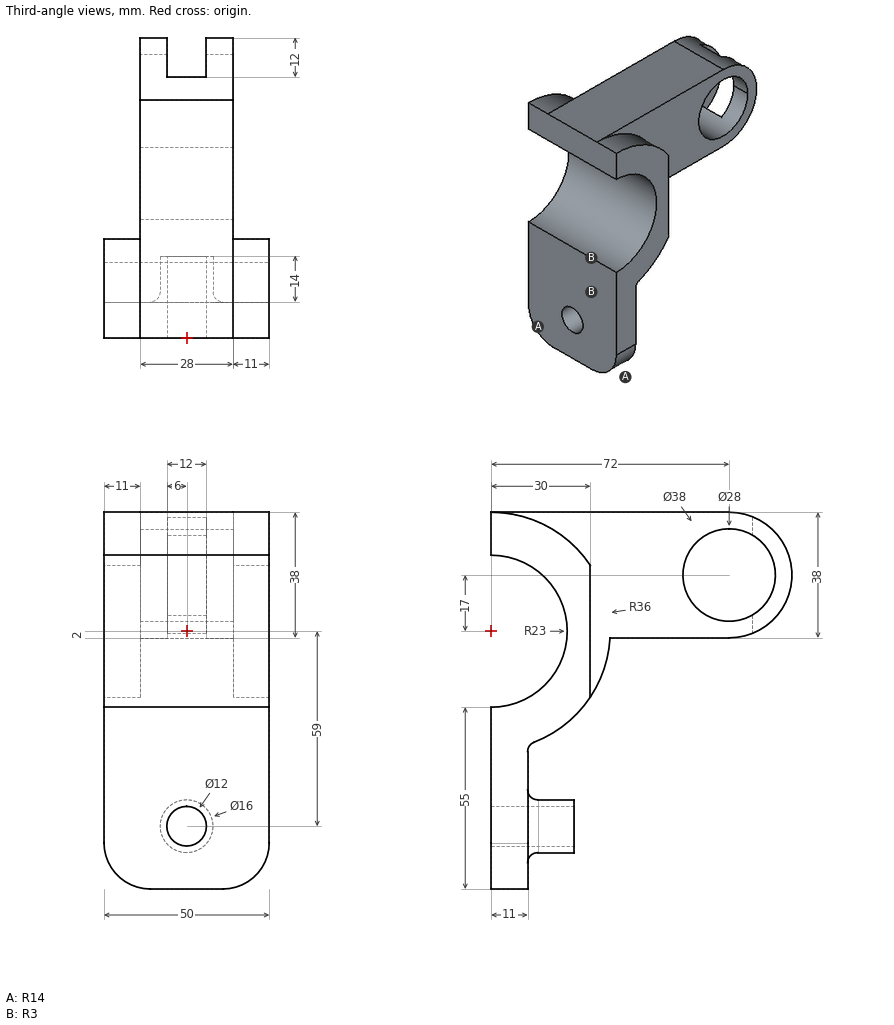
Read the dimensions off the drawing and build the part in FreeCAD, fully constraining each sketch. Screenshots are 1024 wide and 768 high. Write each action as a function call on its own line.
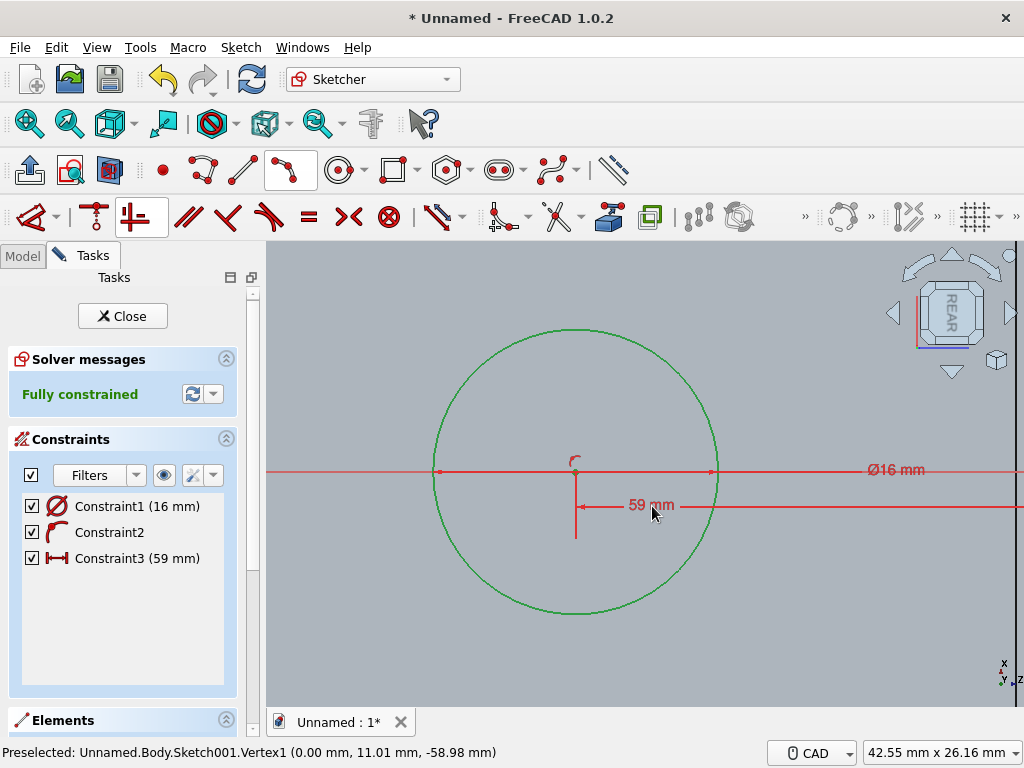
click(123, 316)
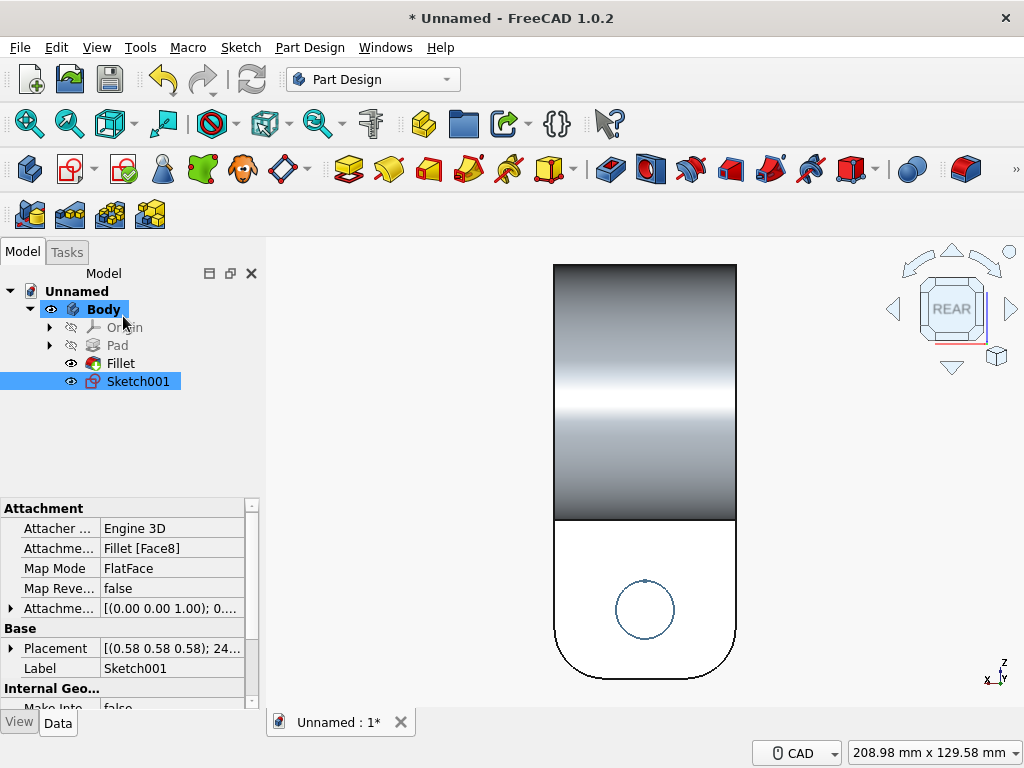
click(350, 170)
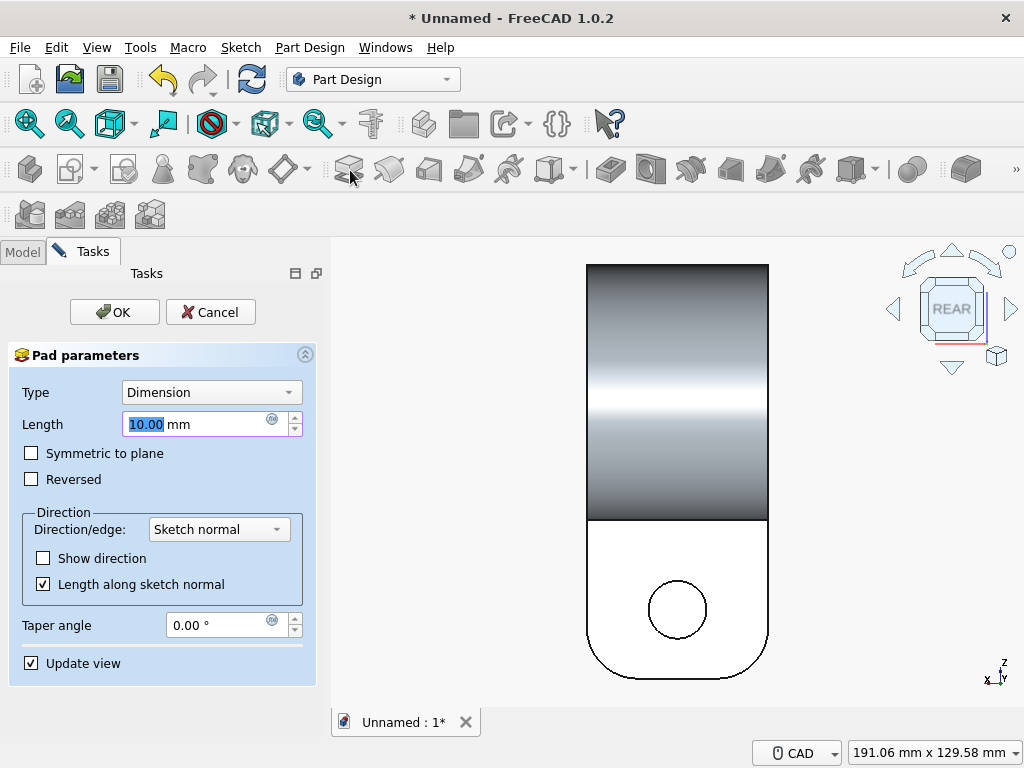
text(14)
key(Tab)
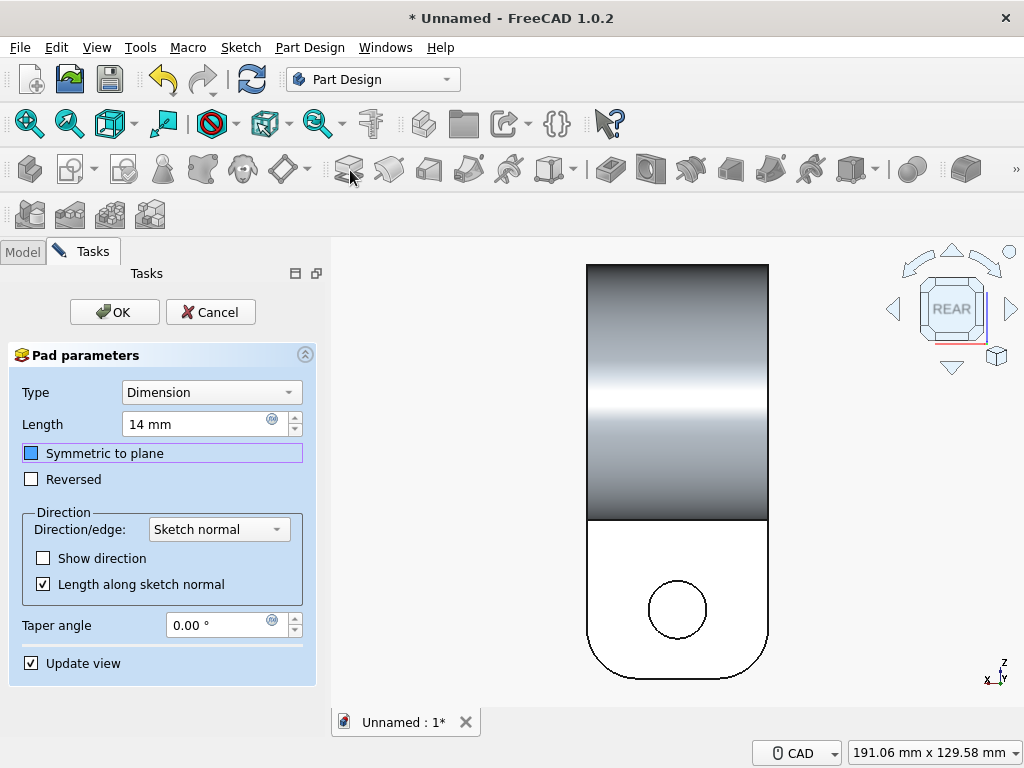
click(115, 312)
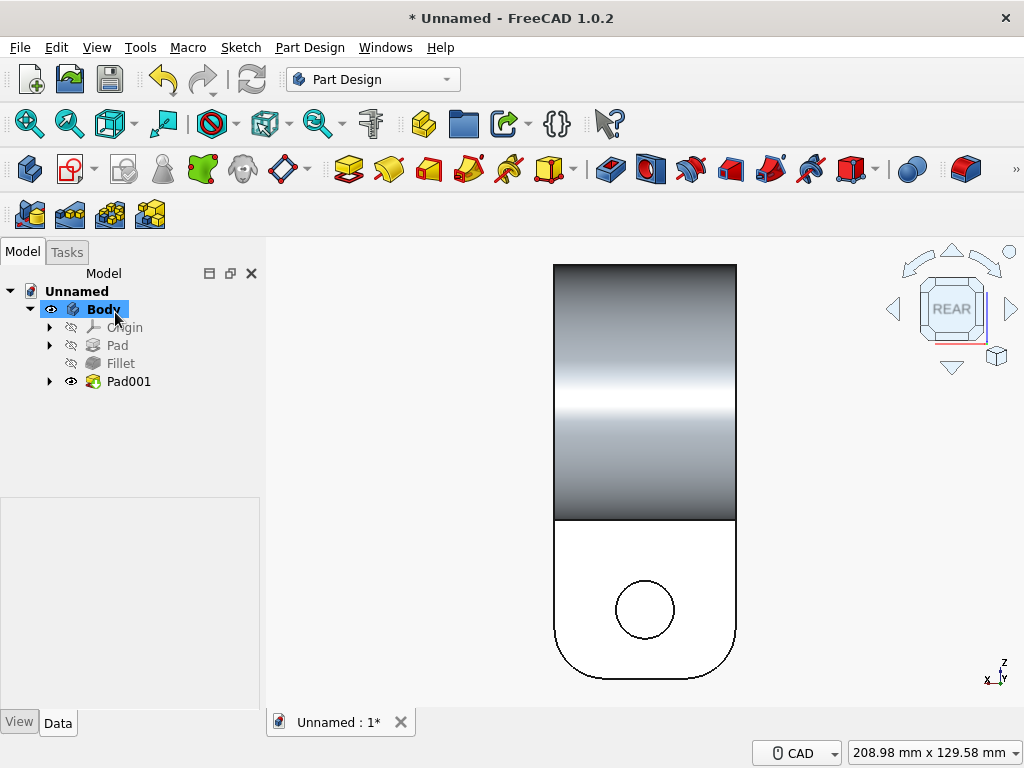
click(645, 609)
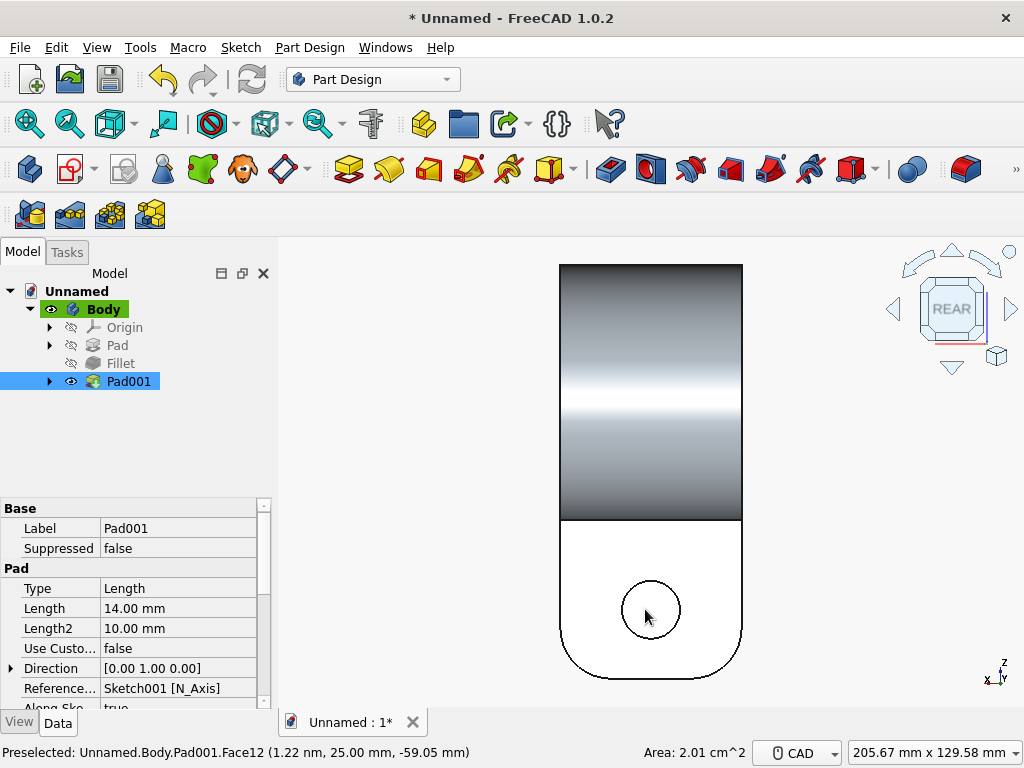
click(70, 170)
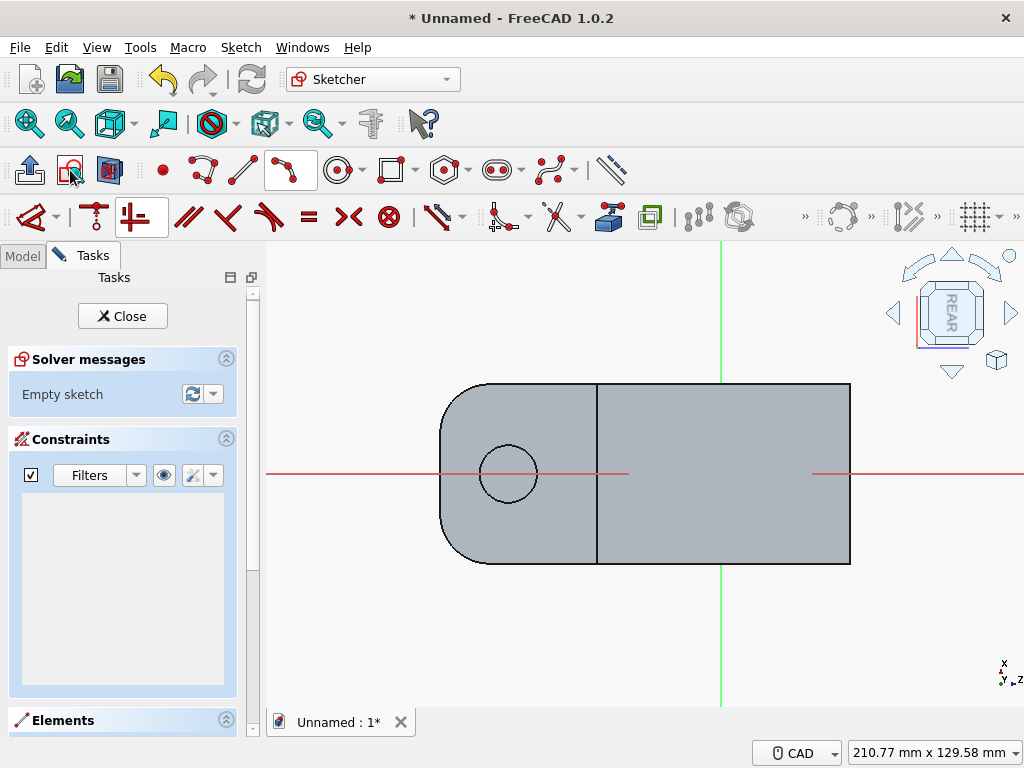
click(110, 170)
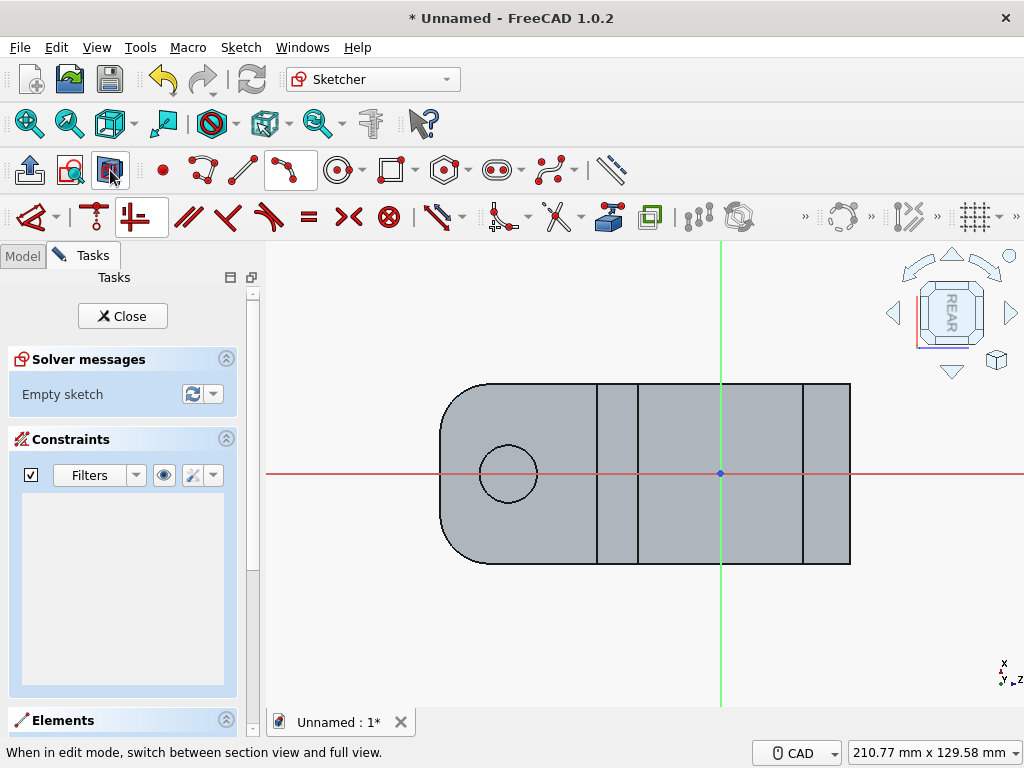
scroll(498, 474, up, 10)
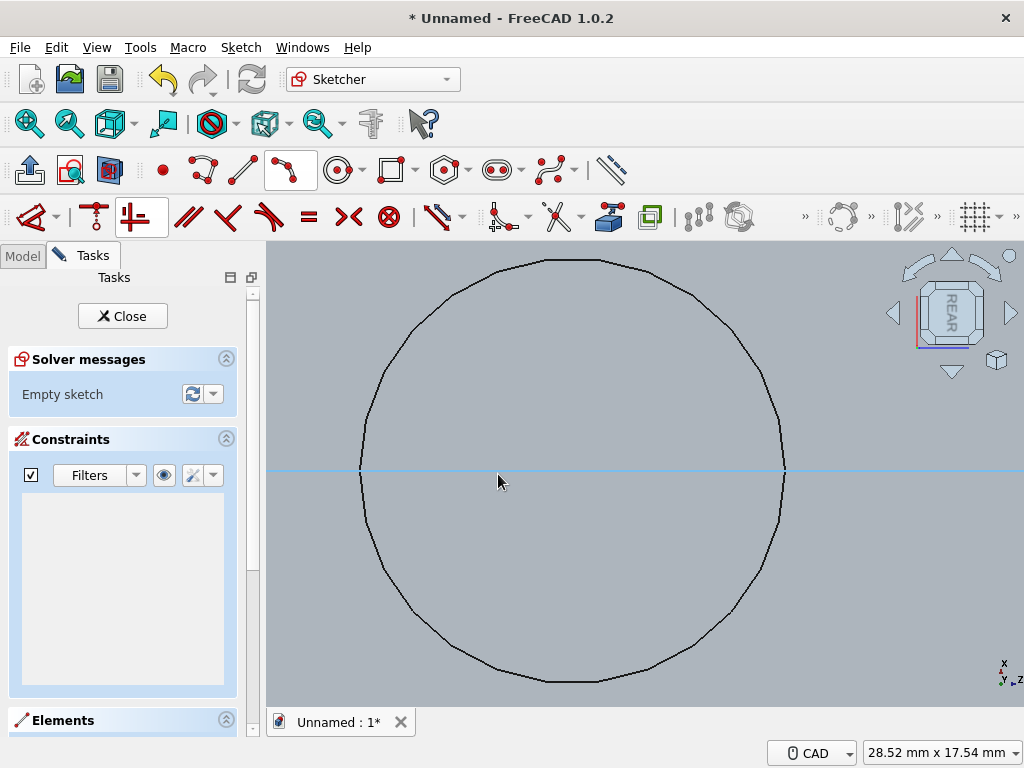
click(338, 170)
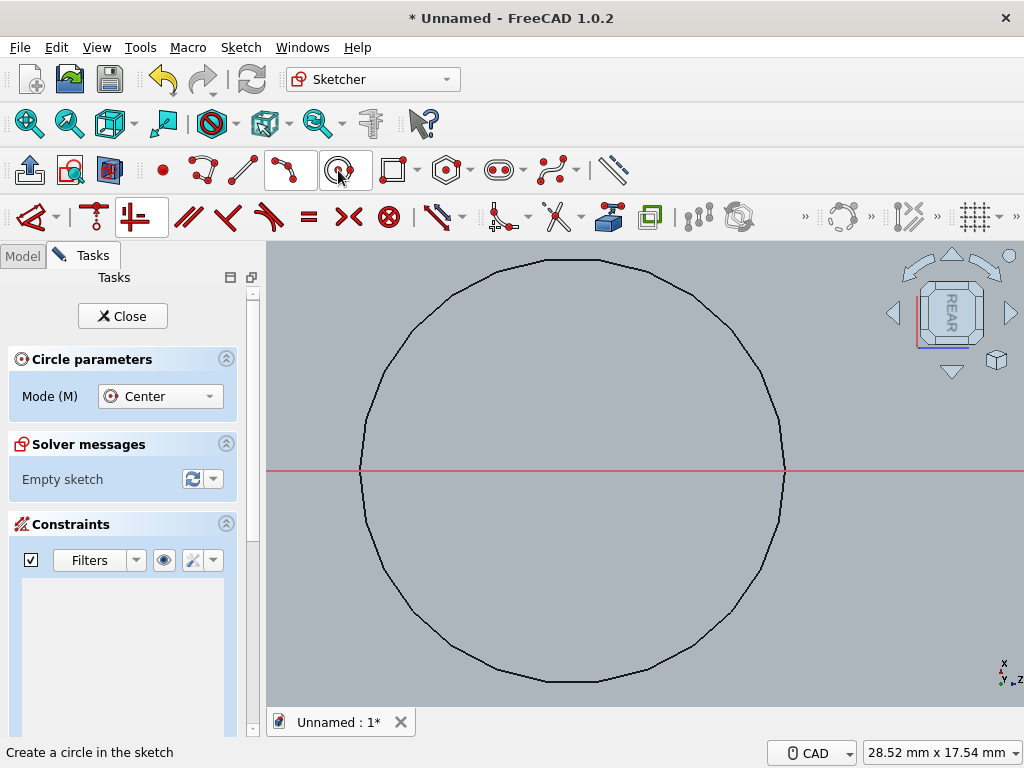
click(572, 471)
move(685, 358)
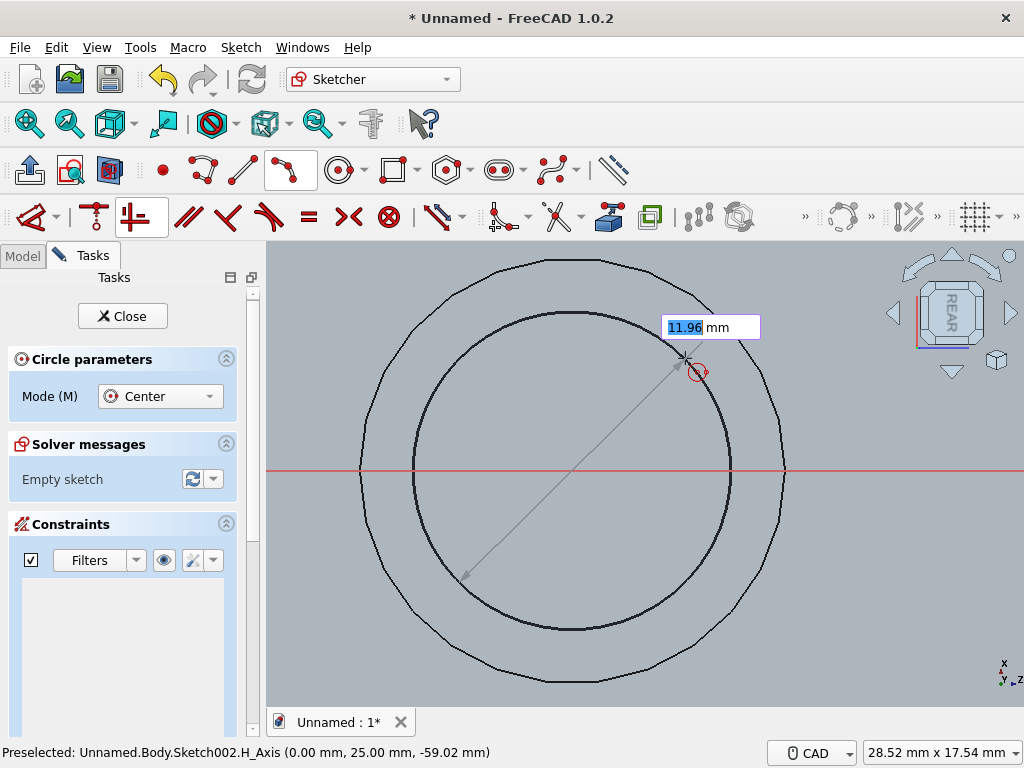
text(12)
key(Return)
key(Escape)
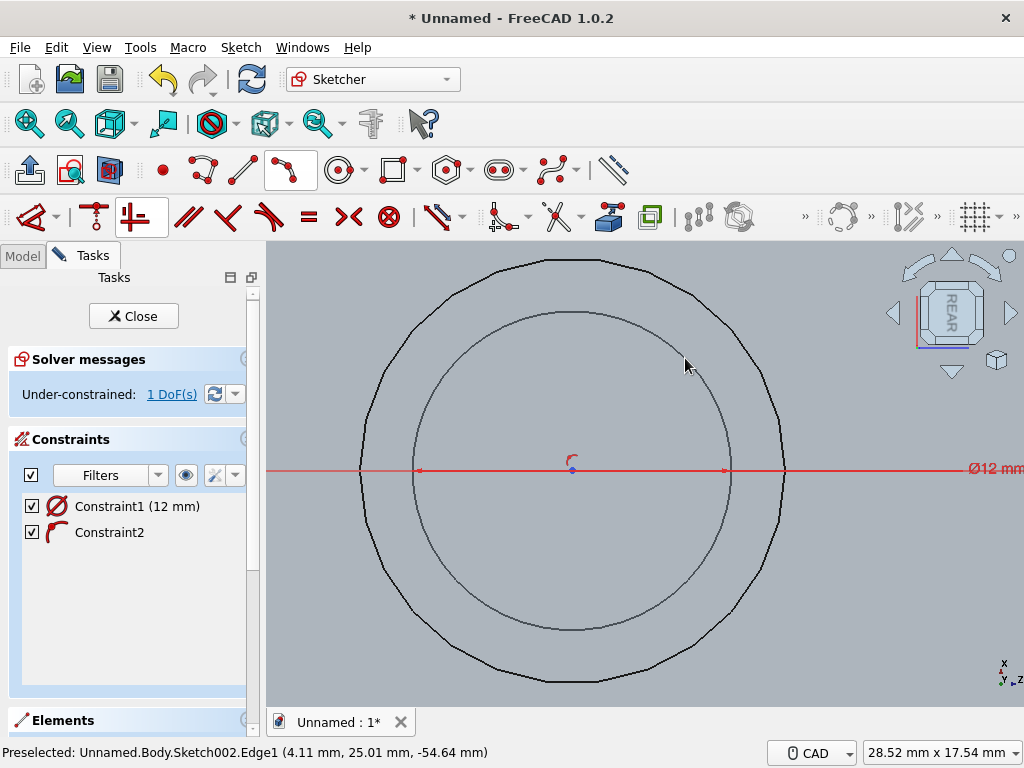
click(32, 218)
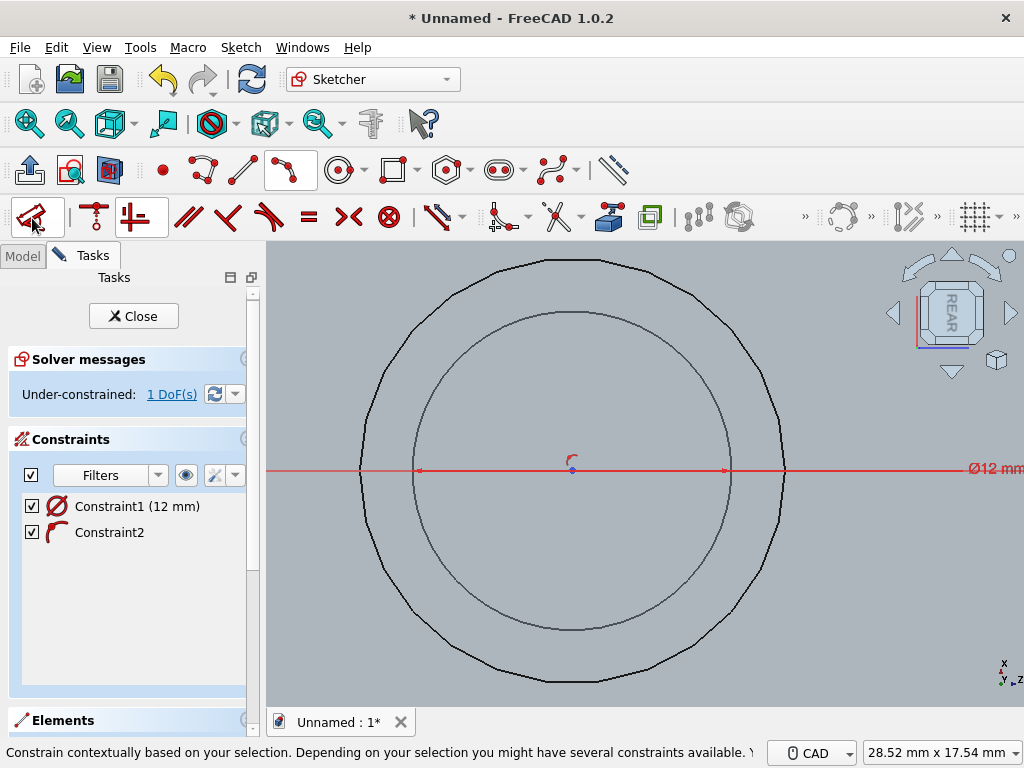
click(572, 471)
click(649, 505)